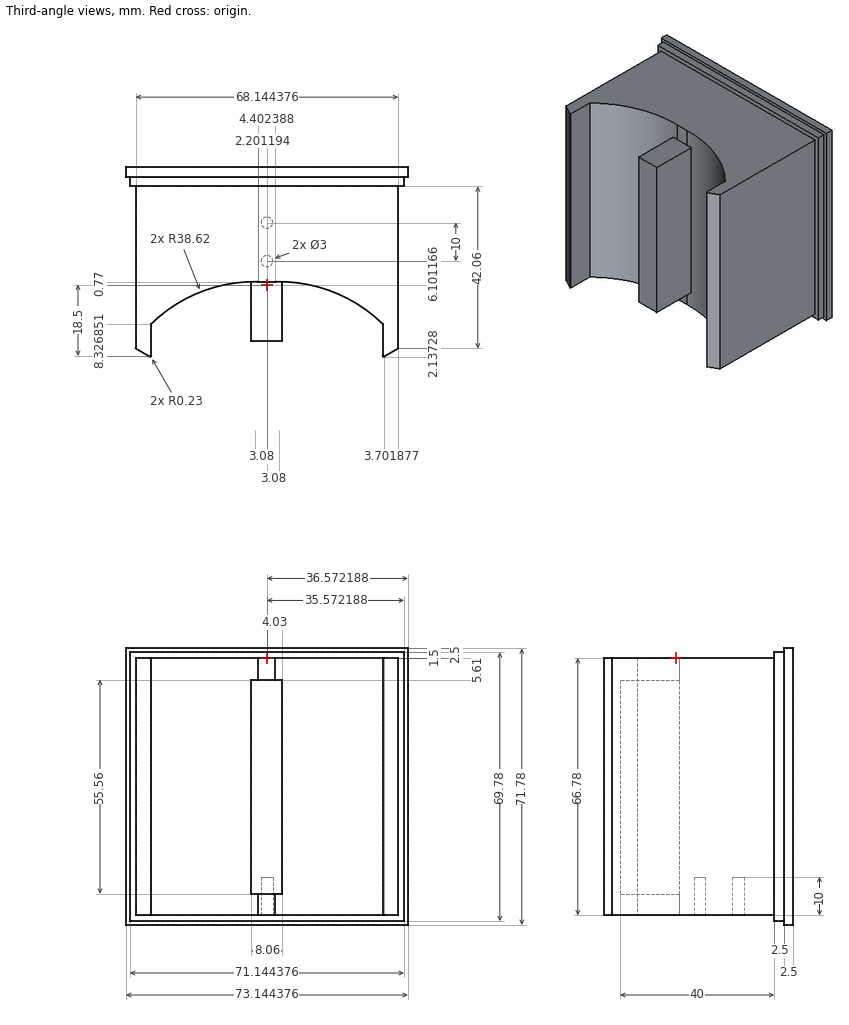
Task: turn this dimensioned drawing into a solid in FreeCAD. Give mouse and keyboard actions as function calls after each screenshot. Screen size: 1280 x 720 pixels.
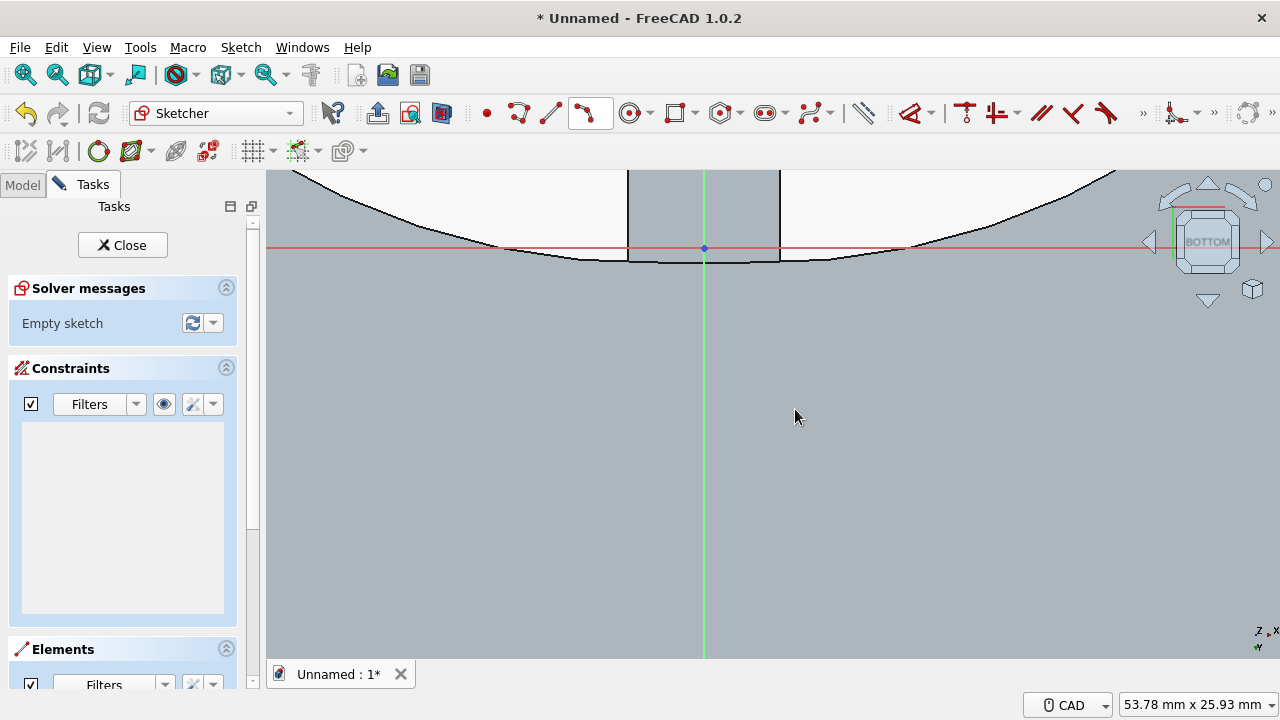
click(630, 114)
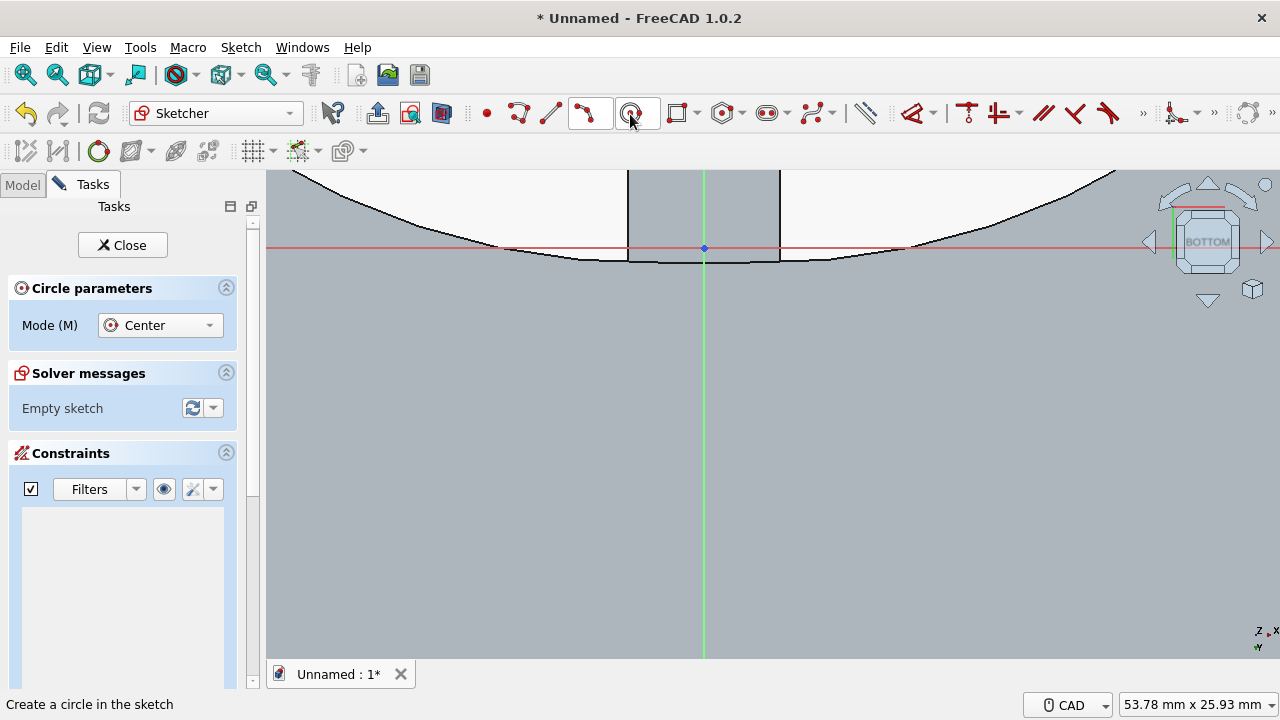
click(704, 363)
move(724, 343)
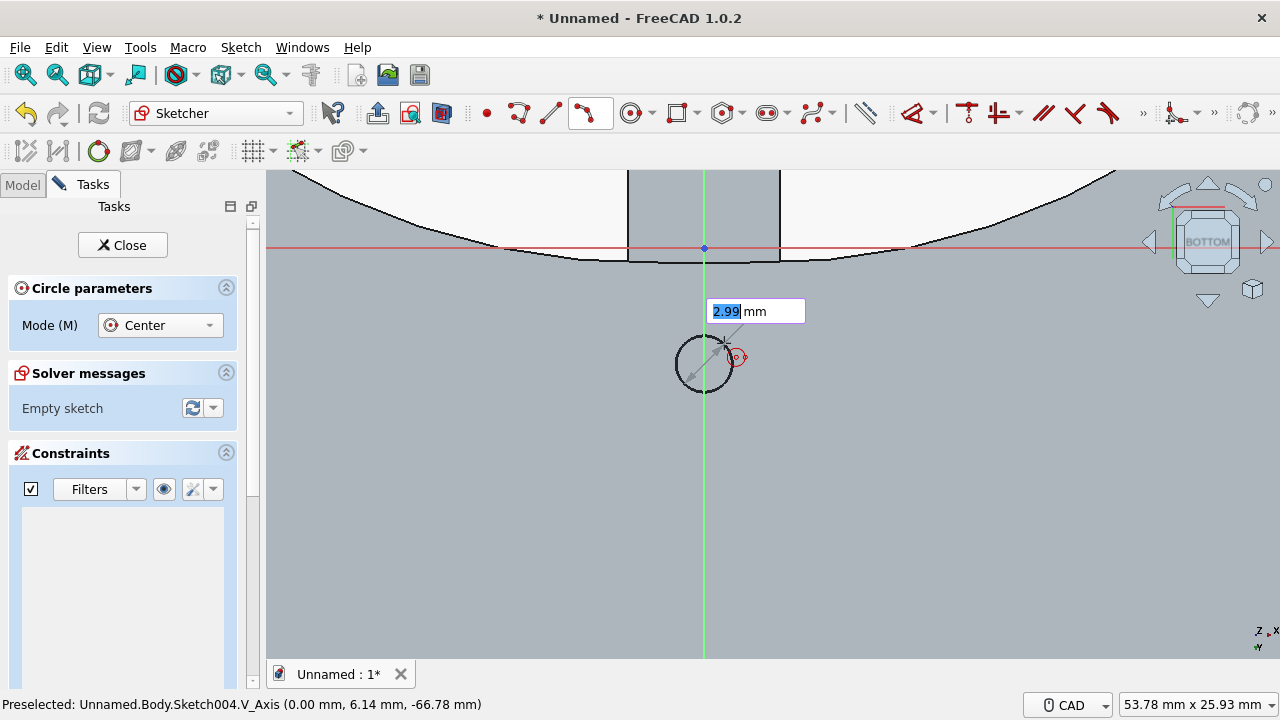
text(3)
key(Return)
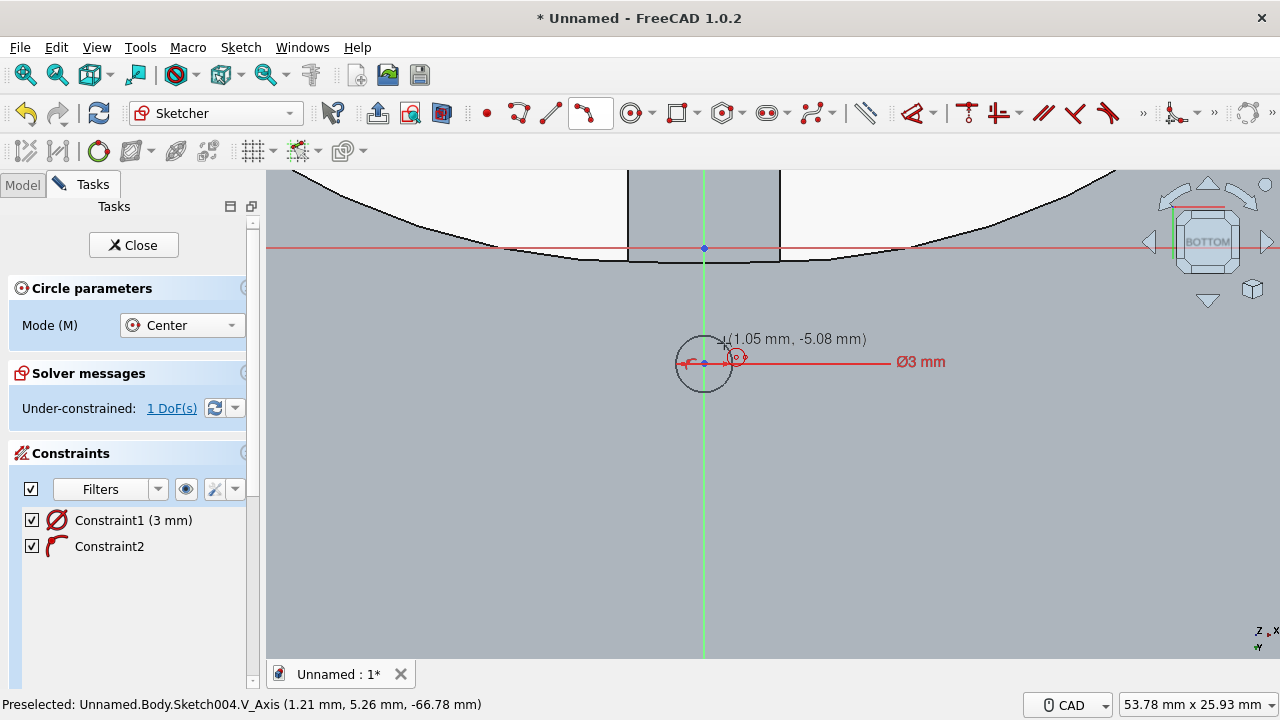
click(704, 552)
move(724, 532)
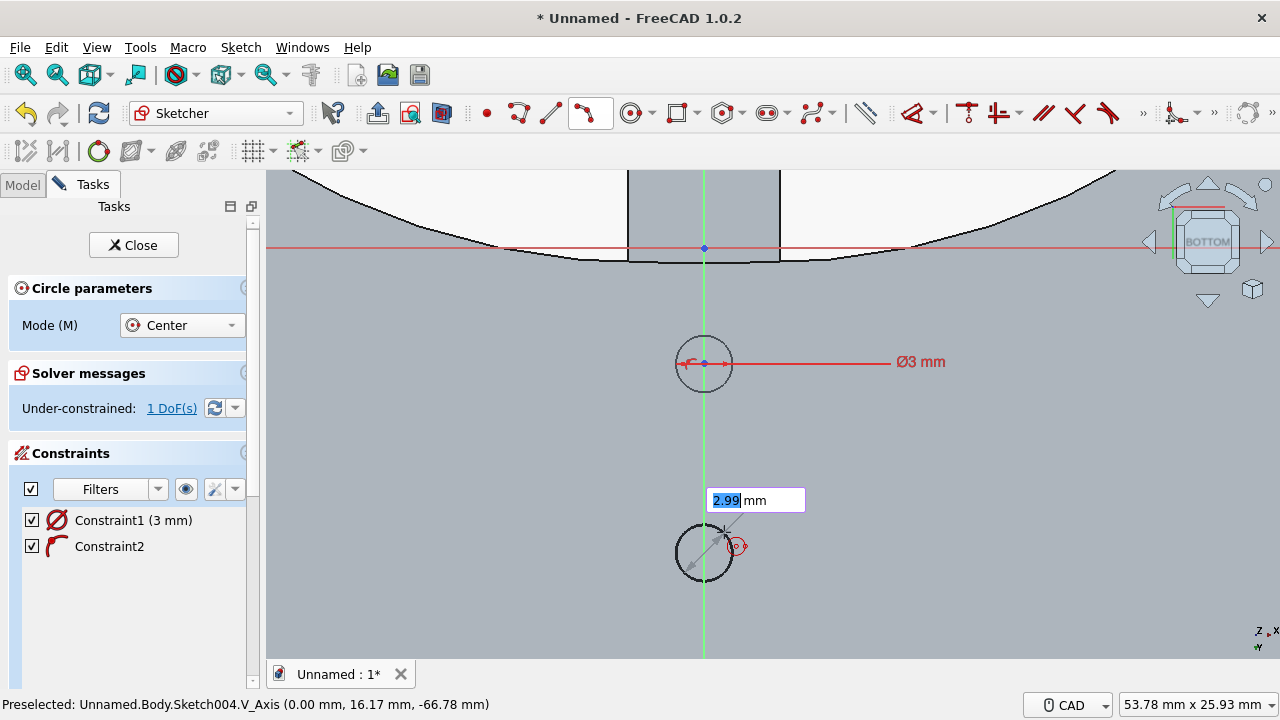
text(3)
key(Return)
key(Escape)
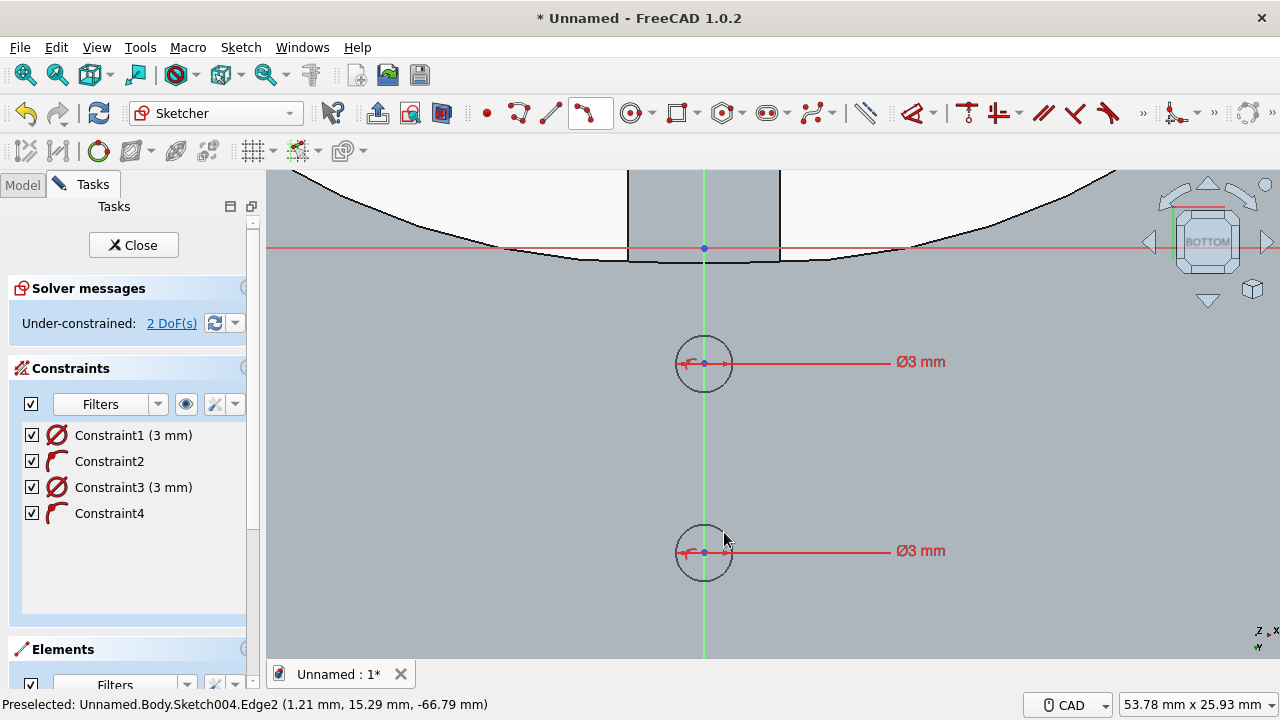
click(912, 114)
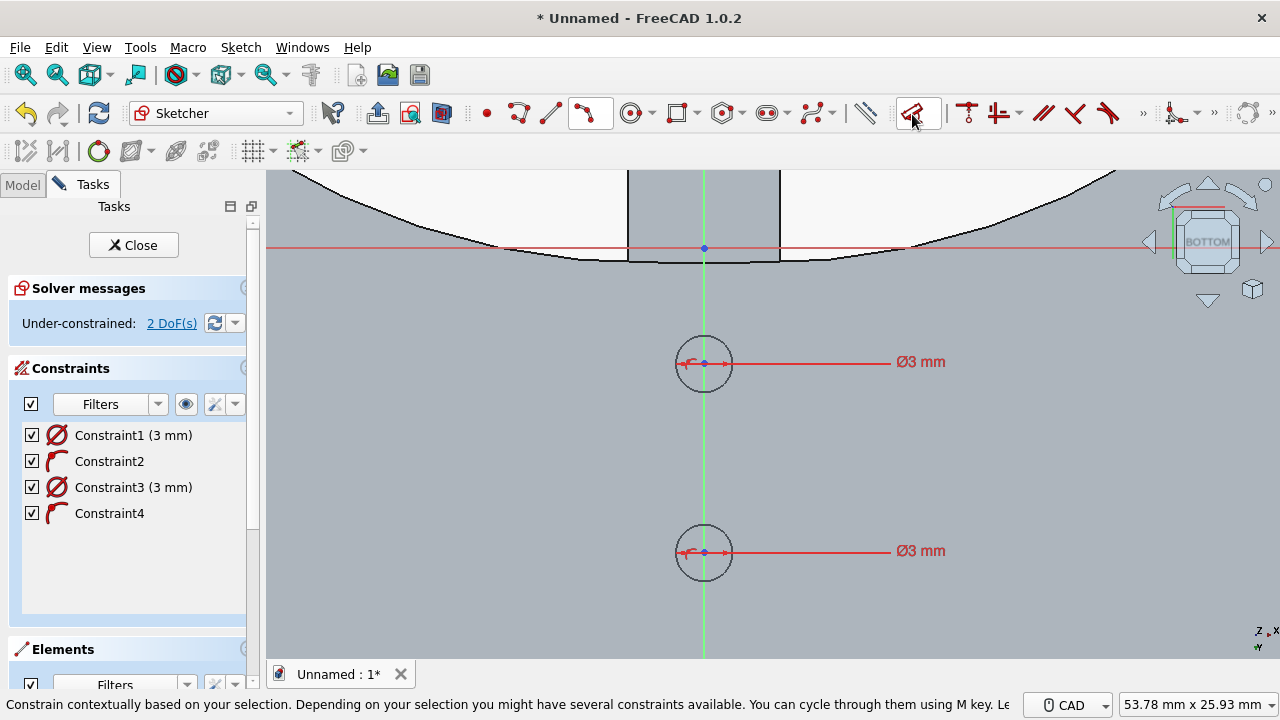
click(704, 364)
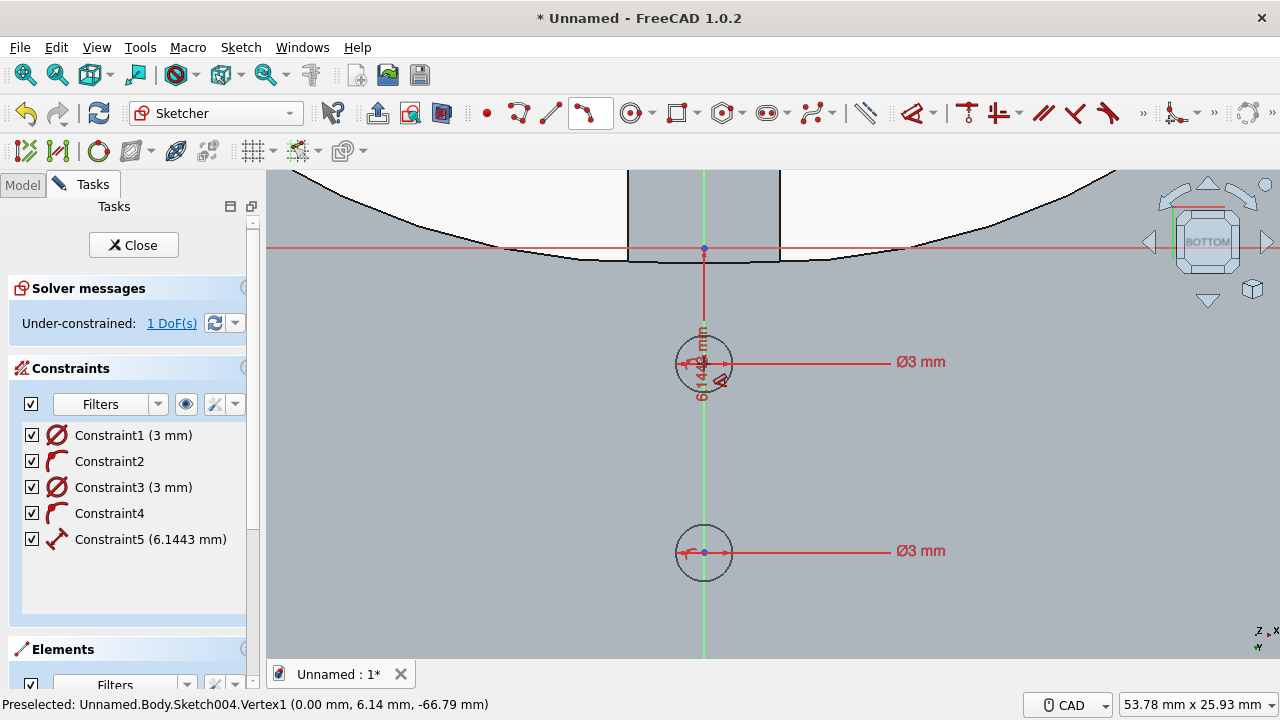
click(704, 553)
click(738, 459)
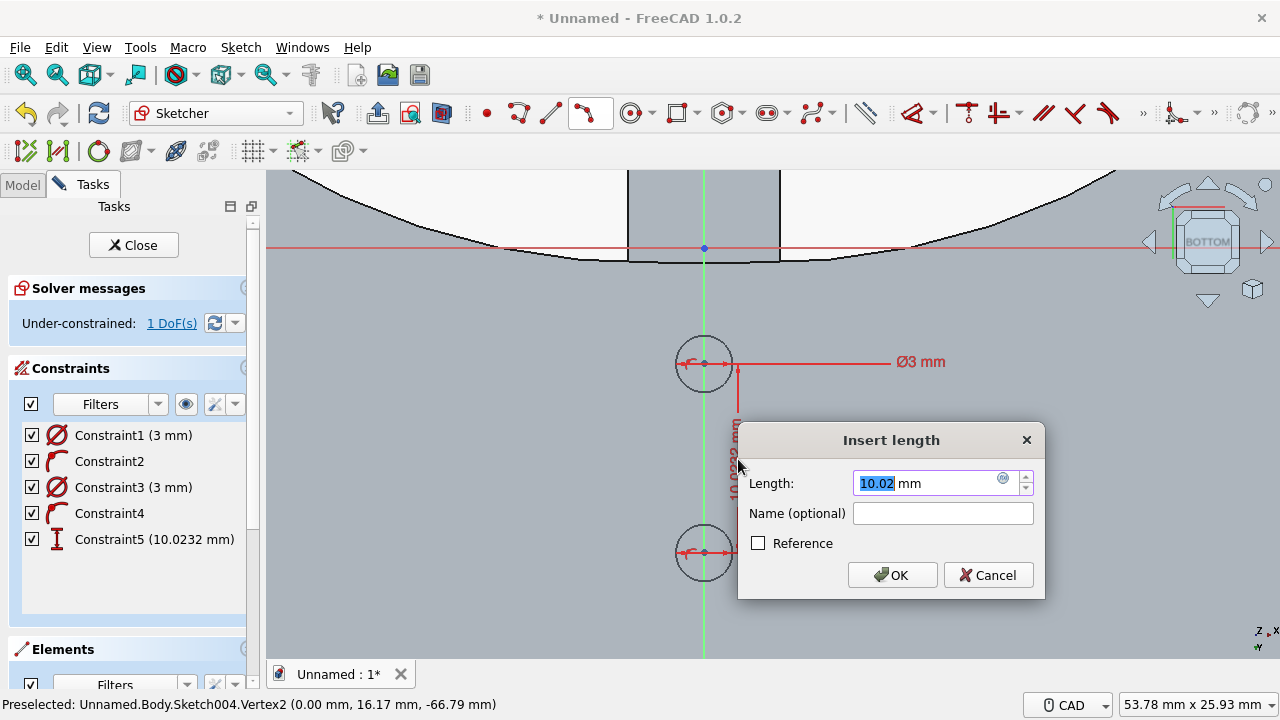
text(10)
key(Return)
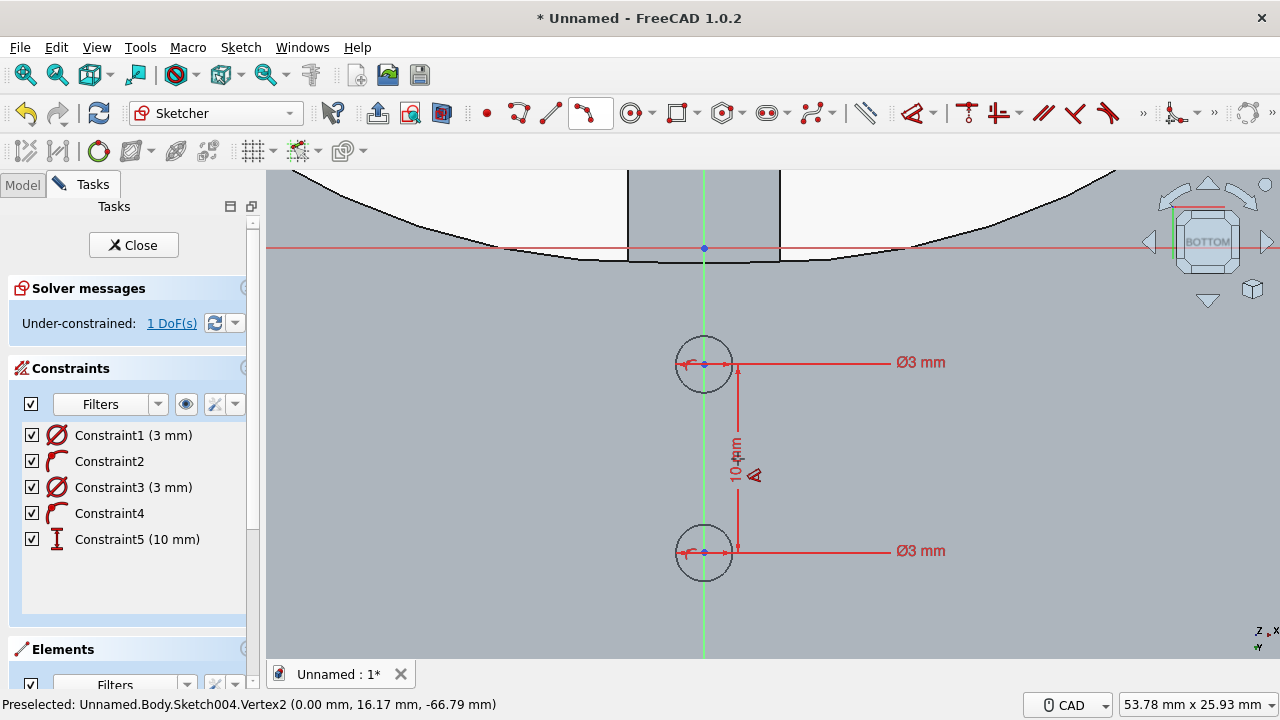
click(704, 364)
click(738, 306)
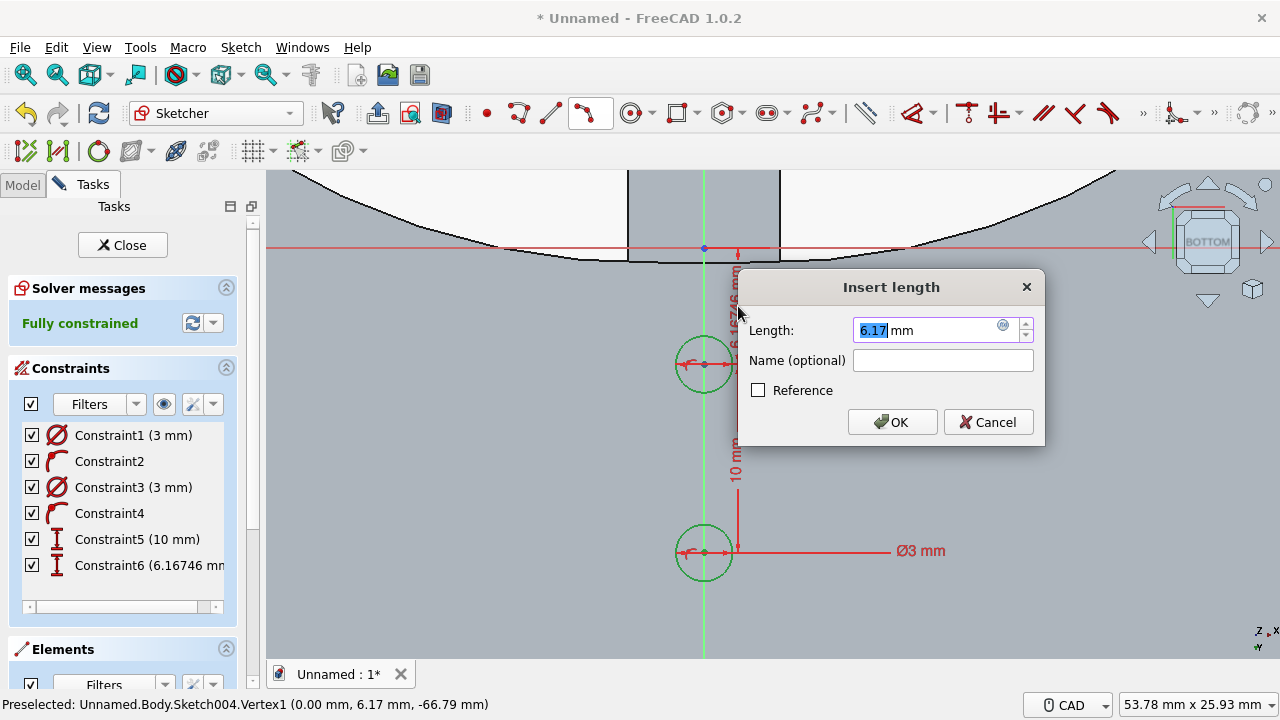
text(6.101166)
key(Return)
key(Escape)